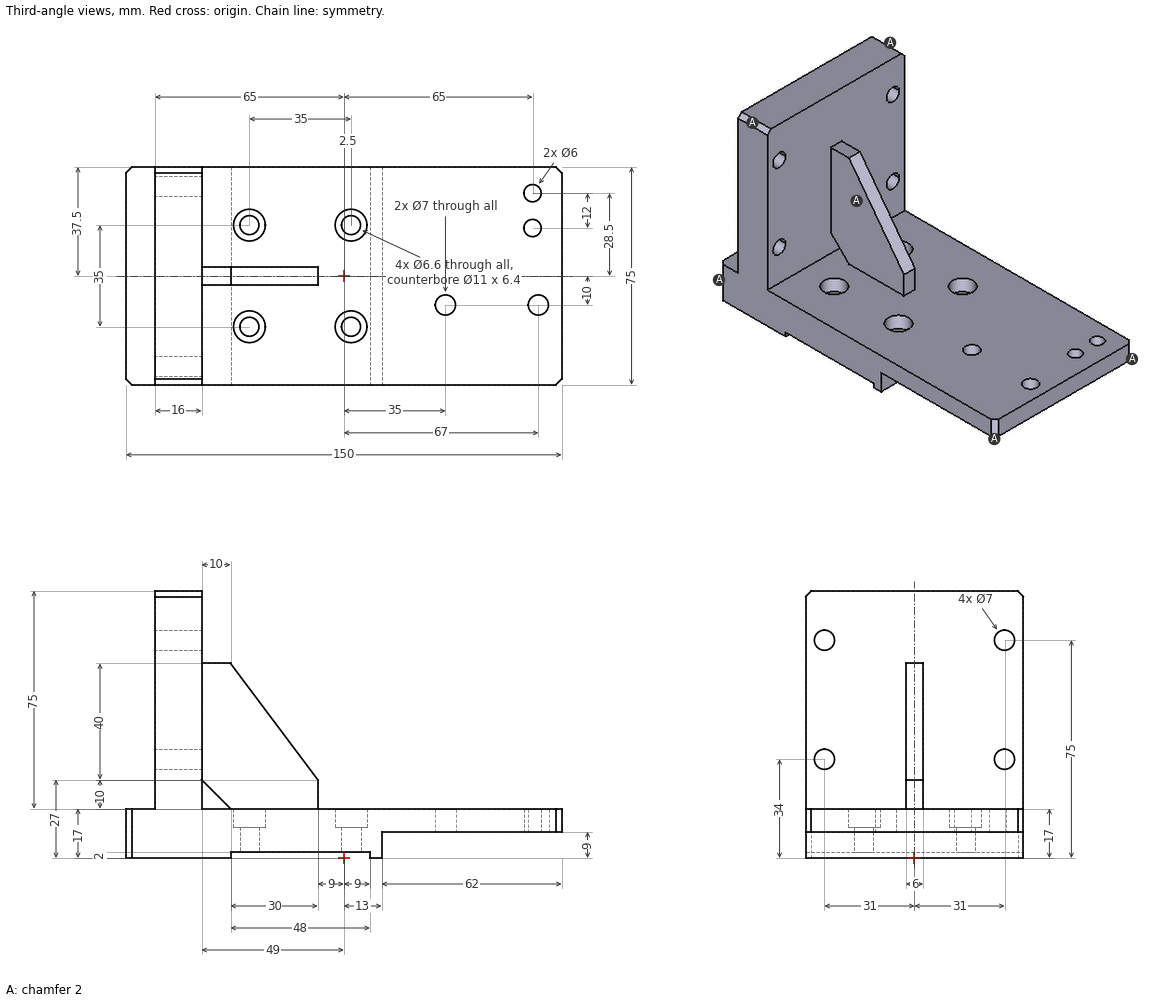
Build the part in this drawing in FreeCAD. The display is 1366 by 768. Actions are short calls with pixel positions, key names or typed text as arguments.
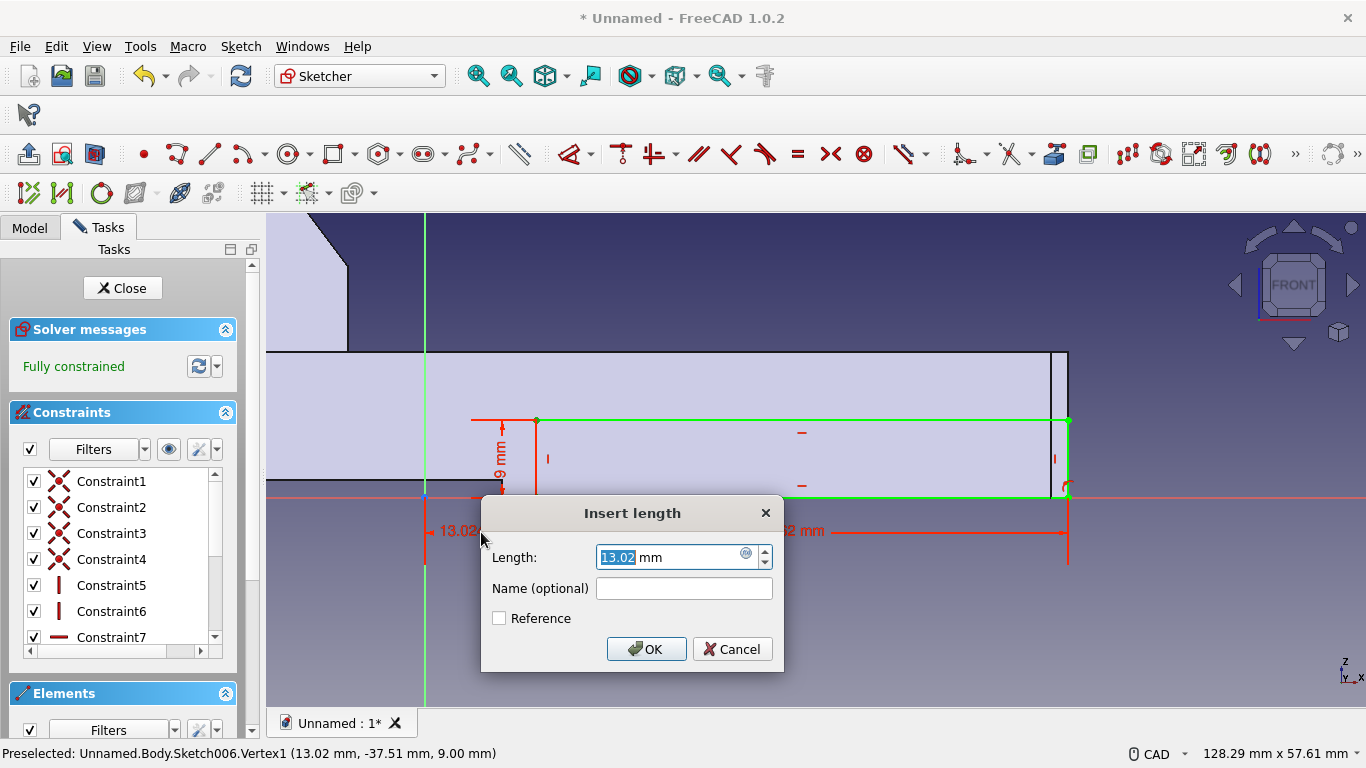
text(13)
key(Return)
key(Escape)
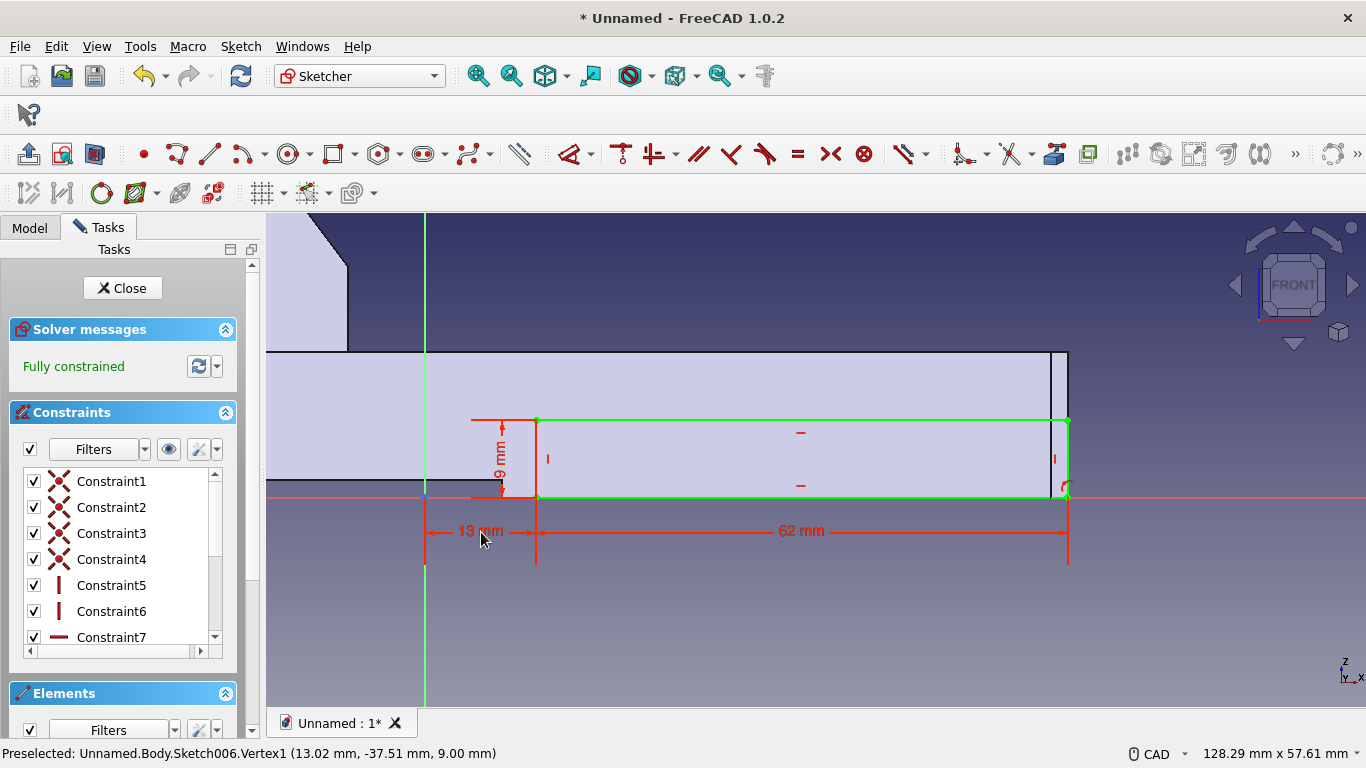
click(123, 288)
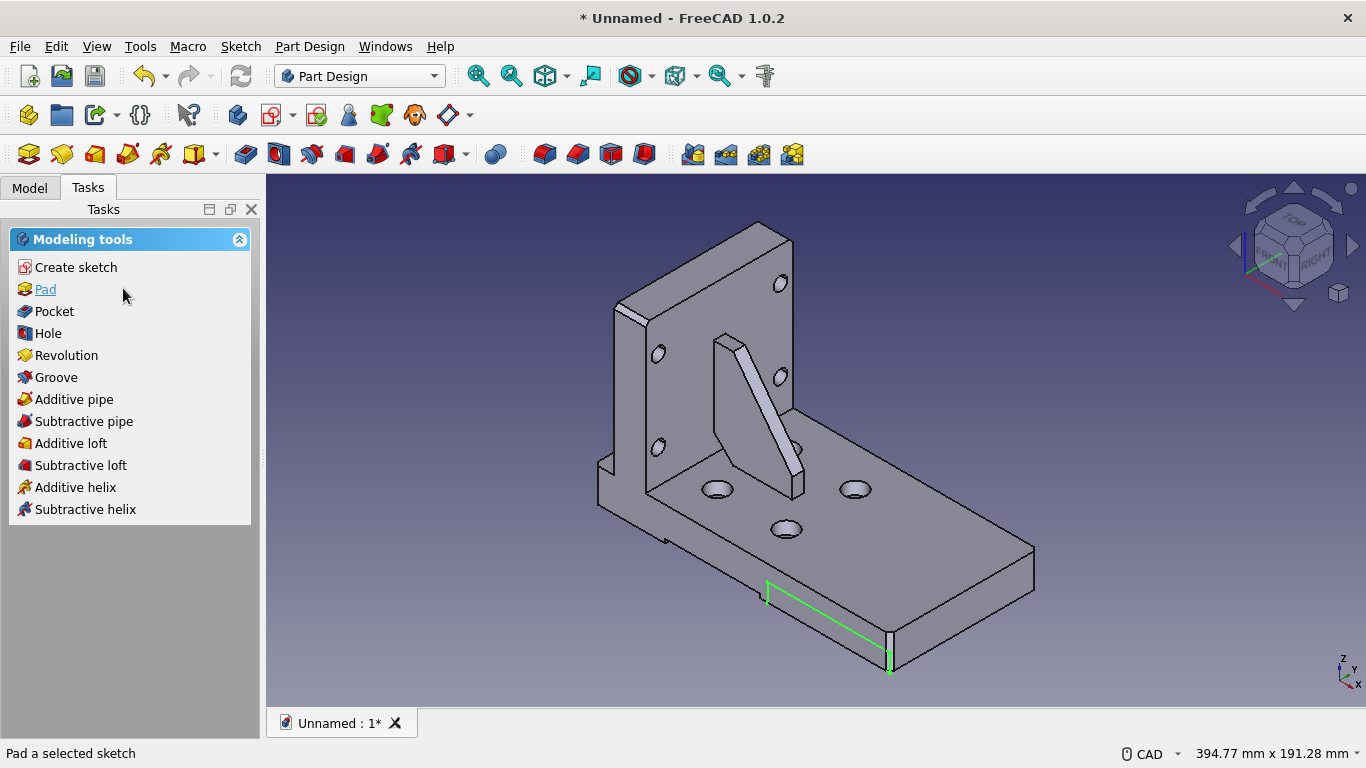
click(246, 154)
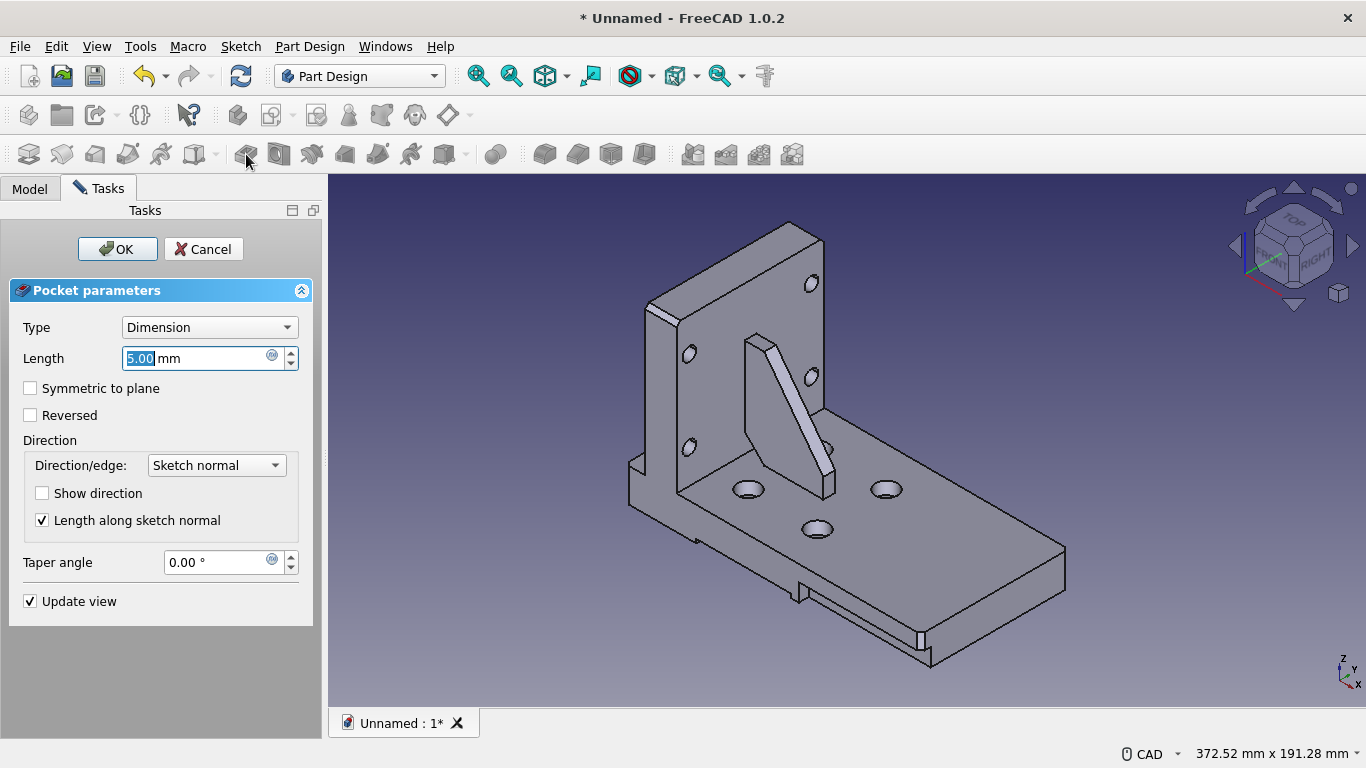
click(210, 328)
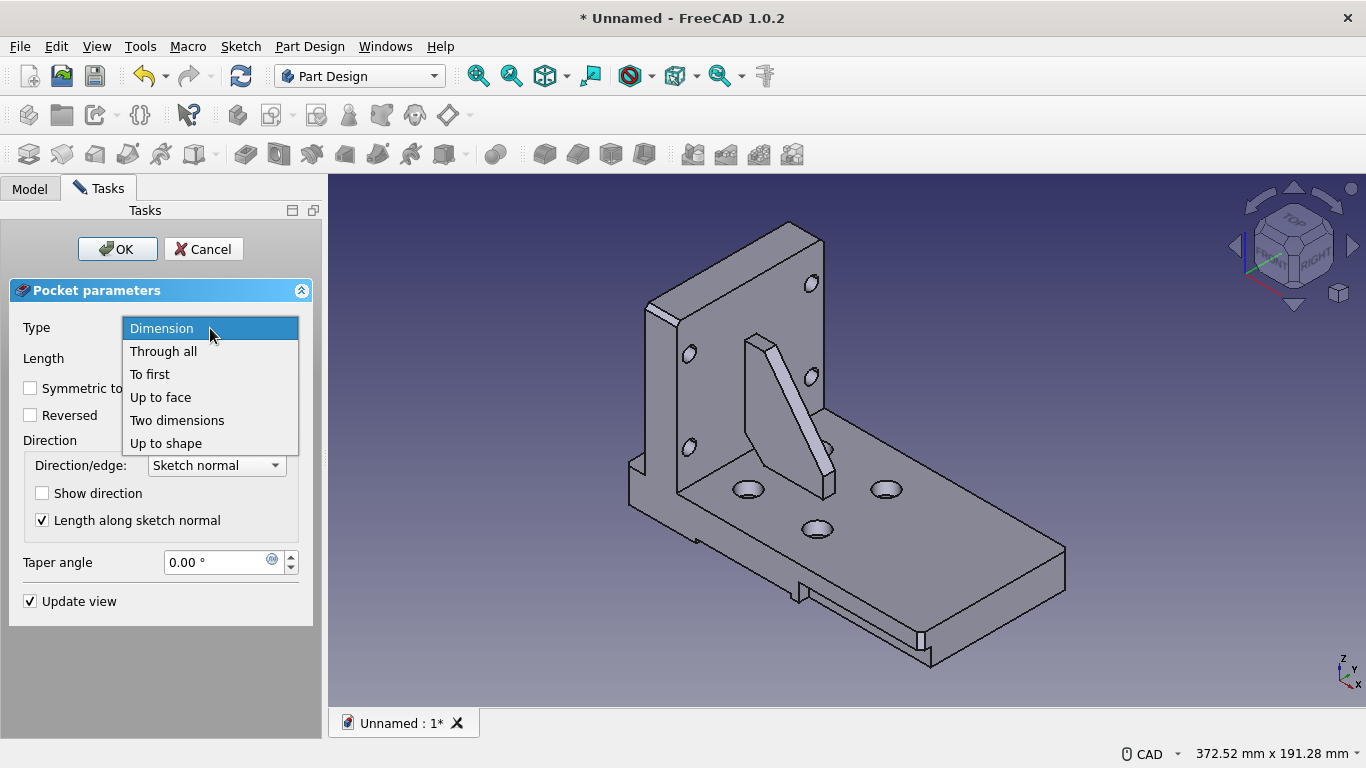
click(208, 352)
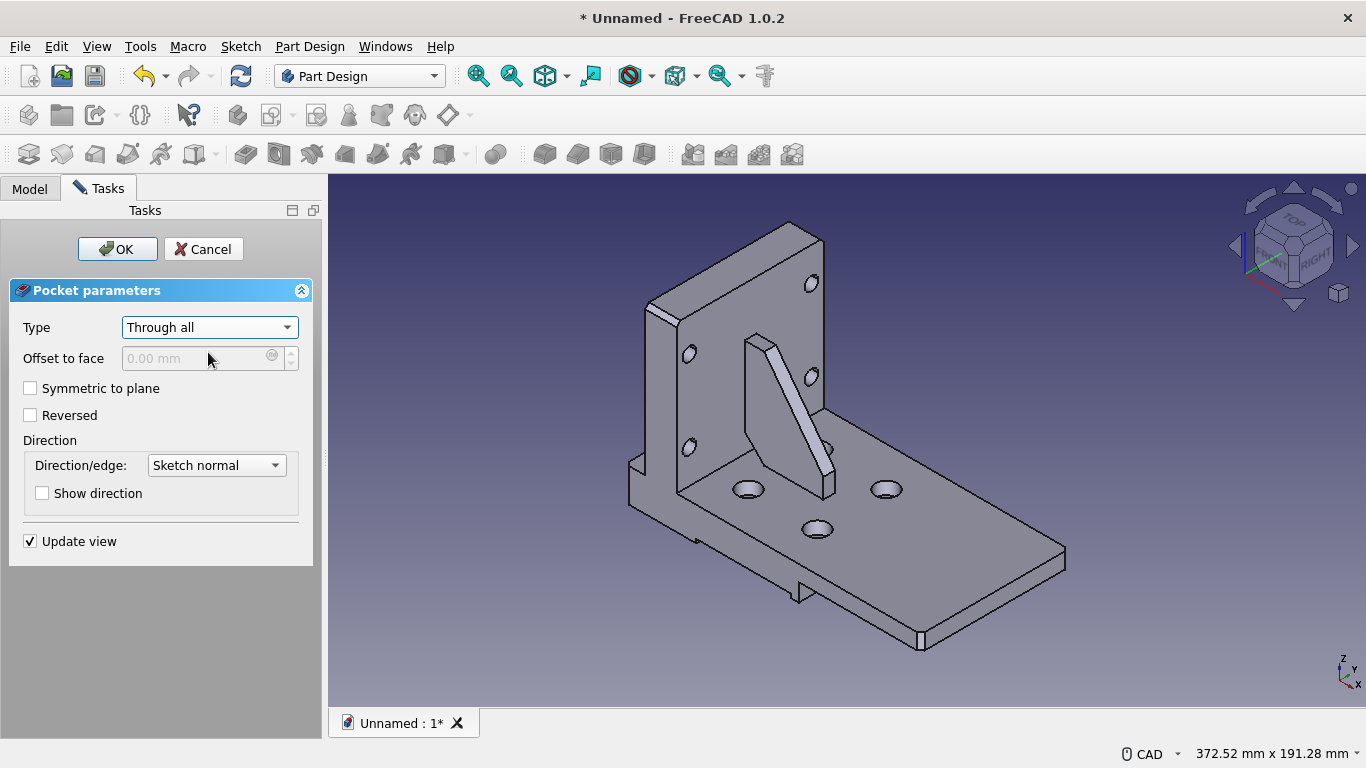
click(118, 249)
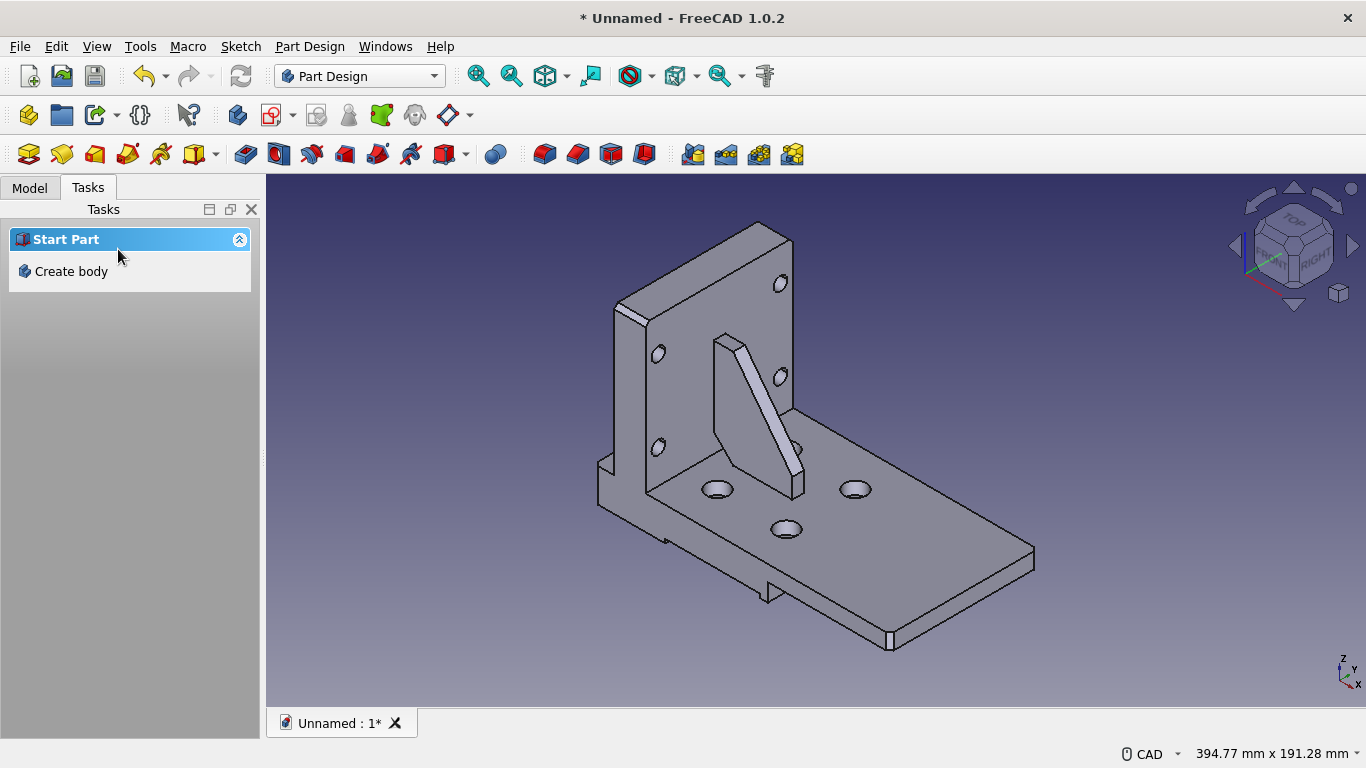
click(877, 540)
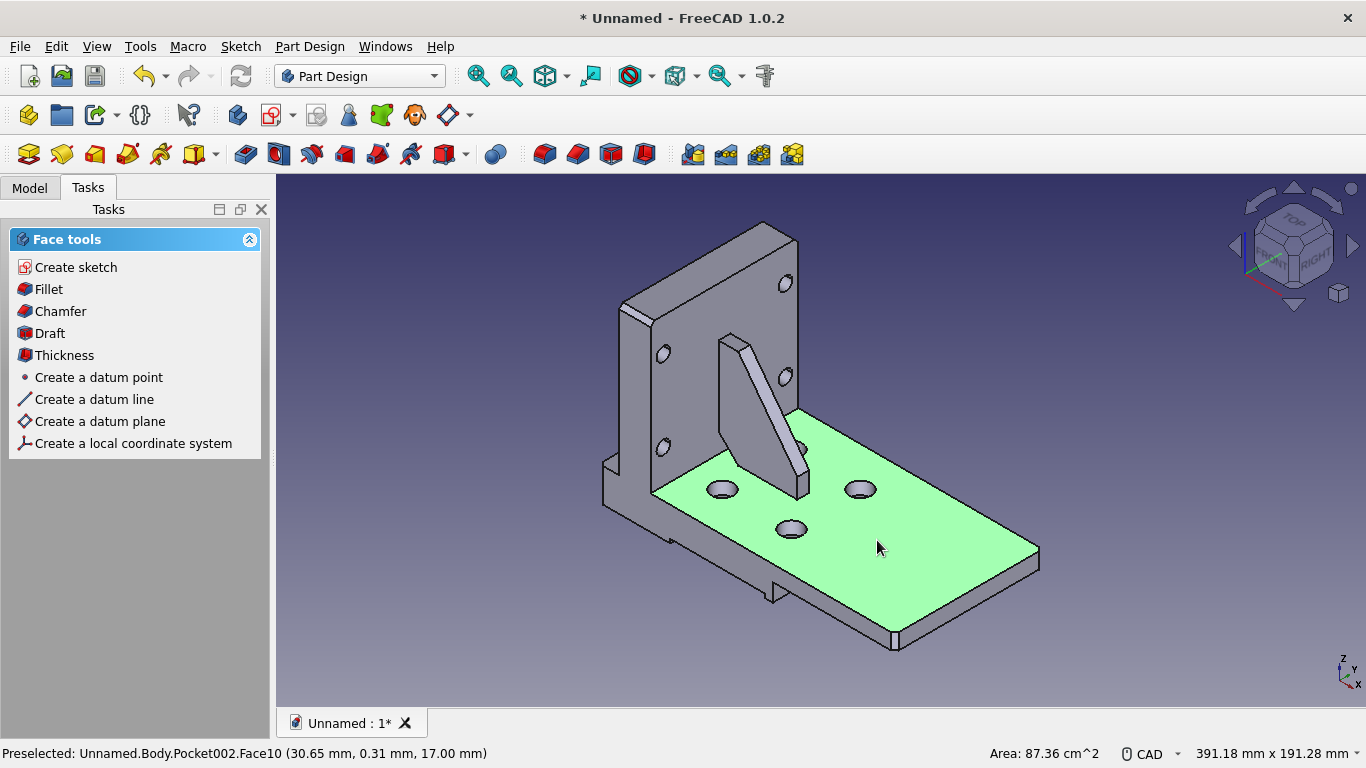
click(270, 116)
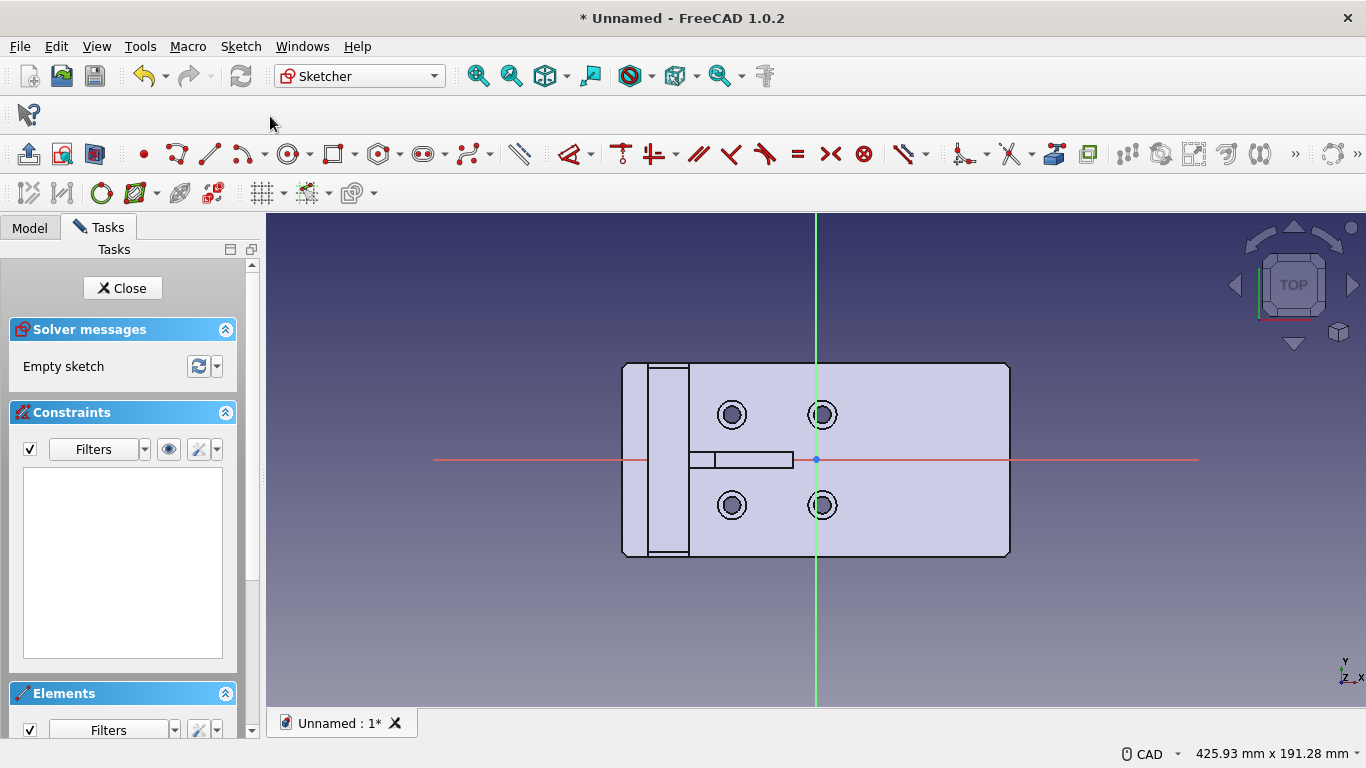
scroll(976, 485, up, 6)